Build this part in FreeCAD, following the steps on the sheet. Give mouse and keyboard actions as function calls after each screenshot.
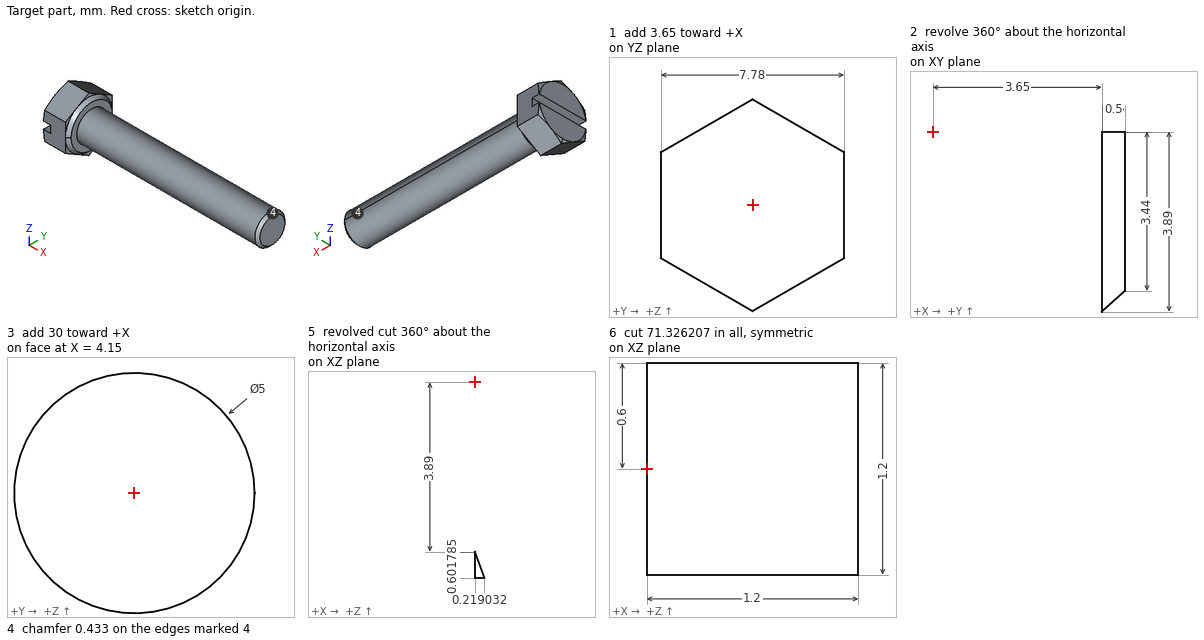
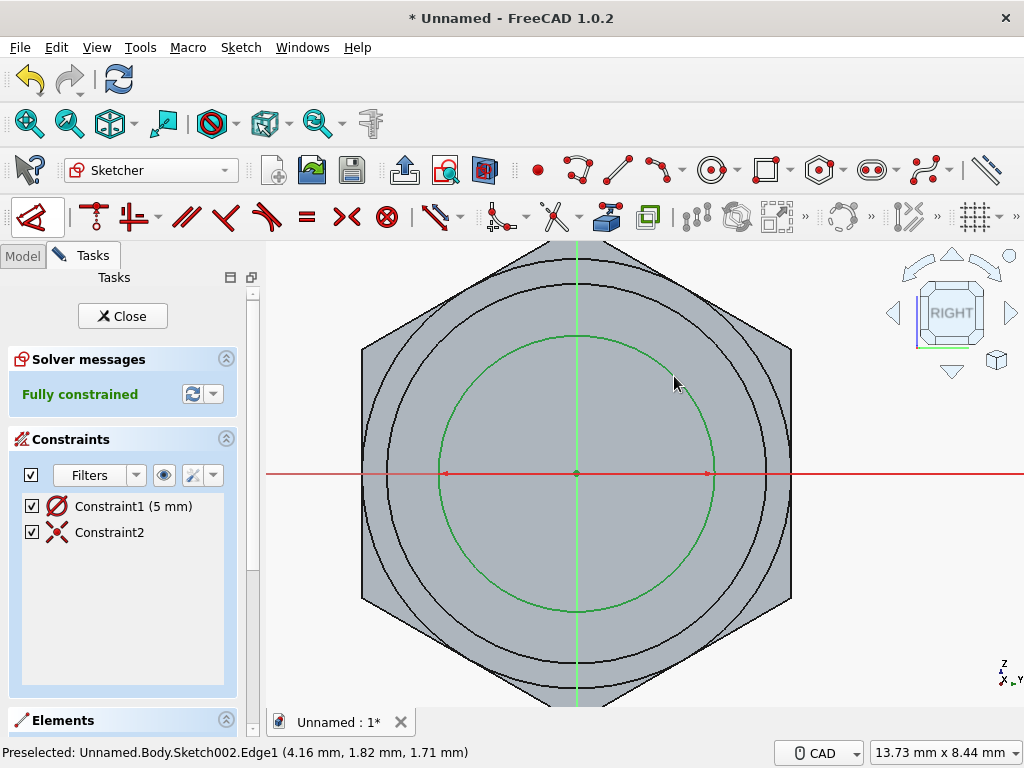
click(123, 316)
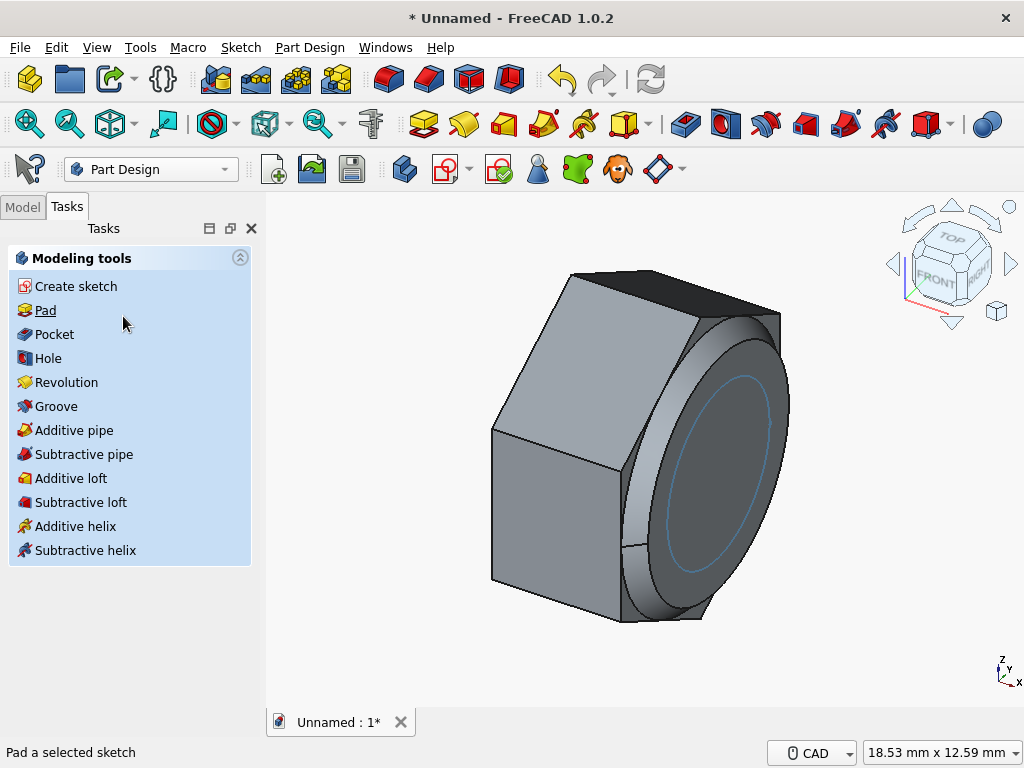
click(424, 124)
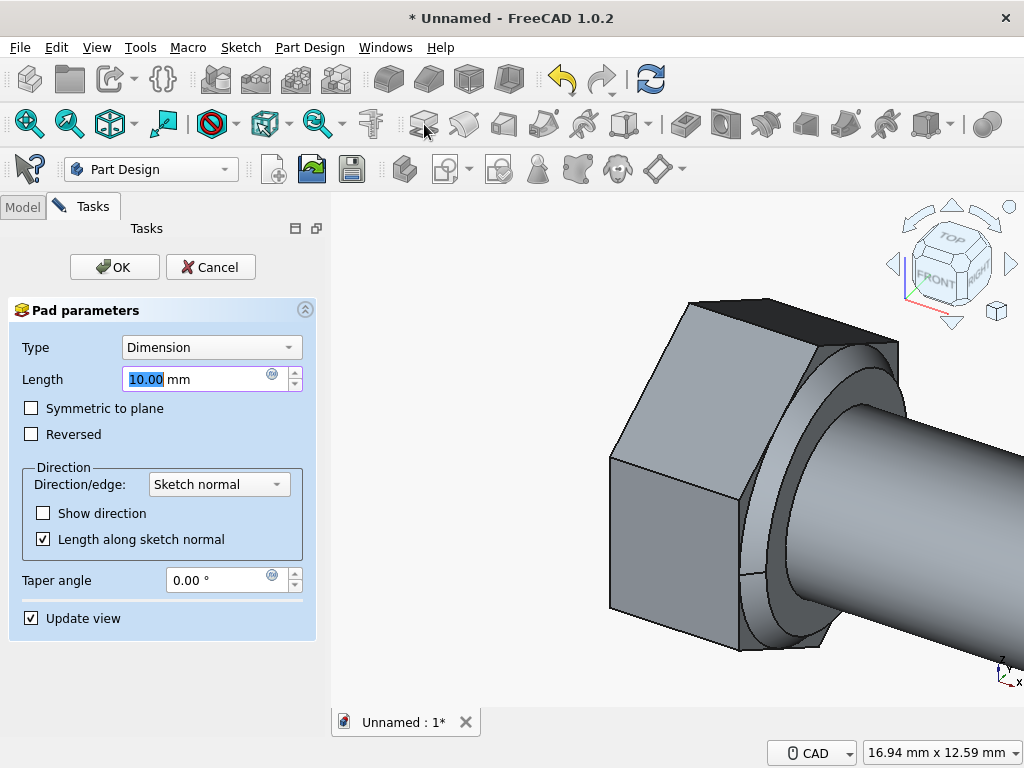
text(30)
key(Tab)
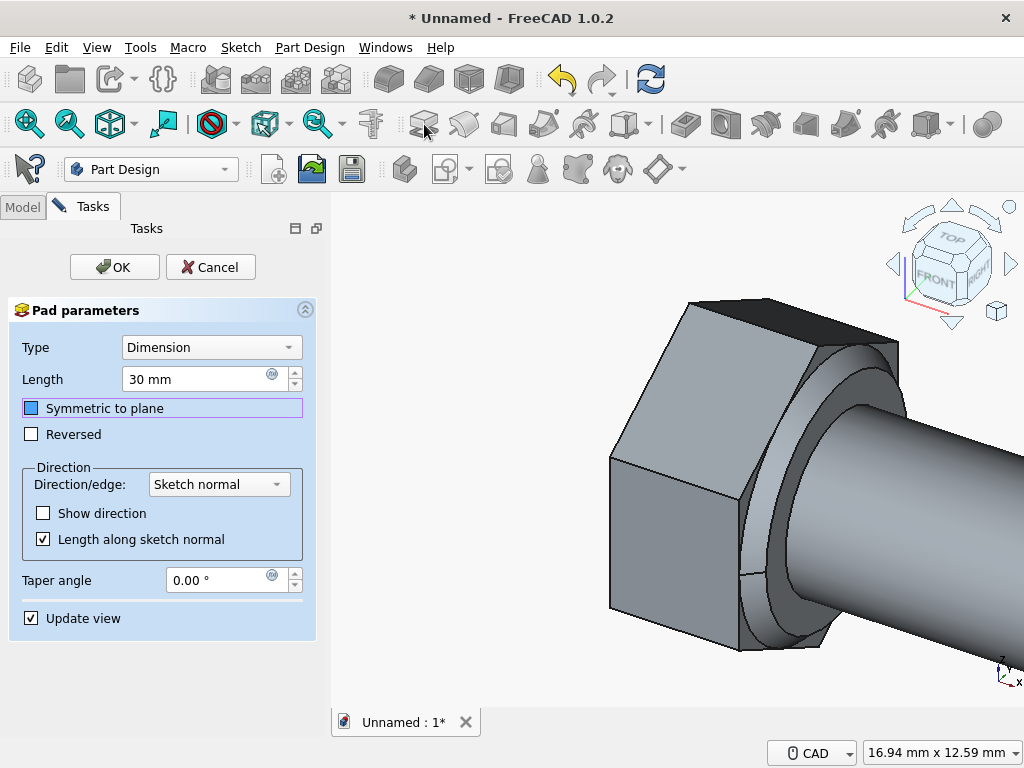
click(115, 267)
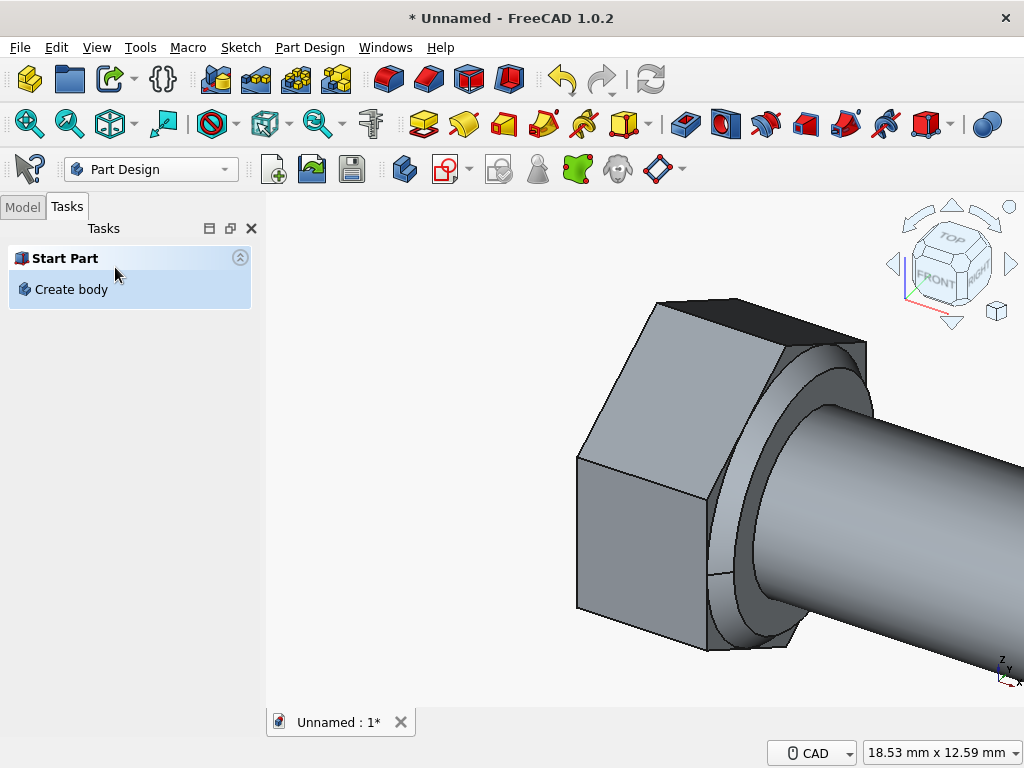
key(v)
key(f)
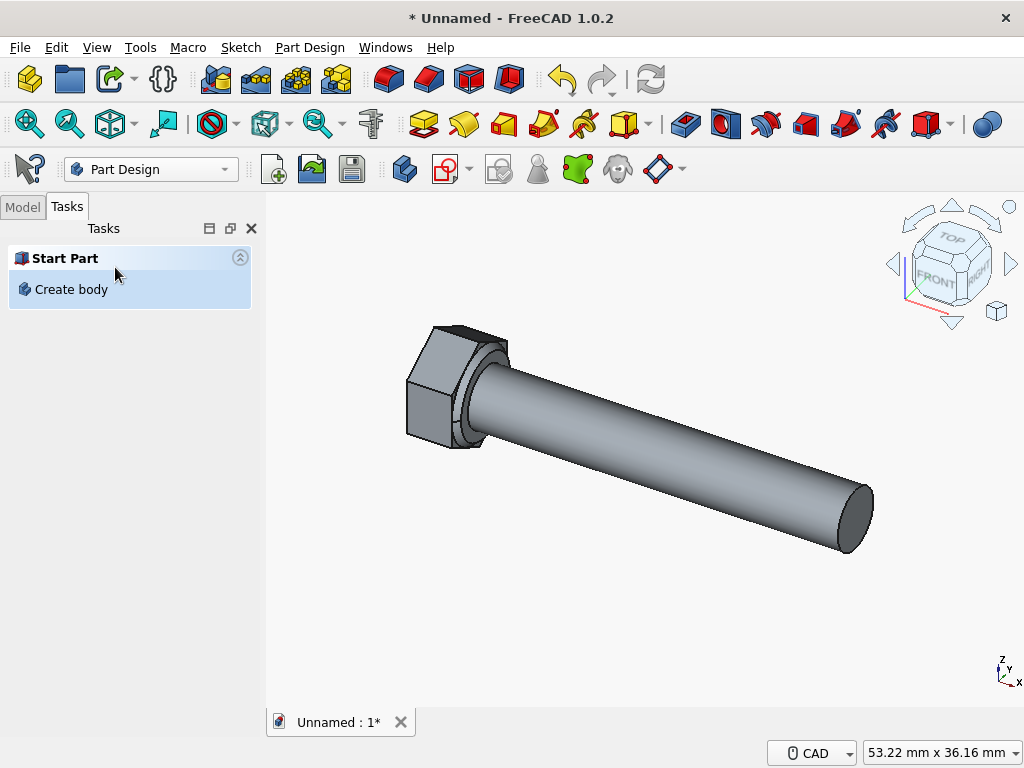
click(838, 536)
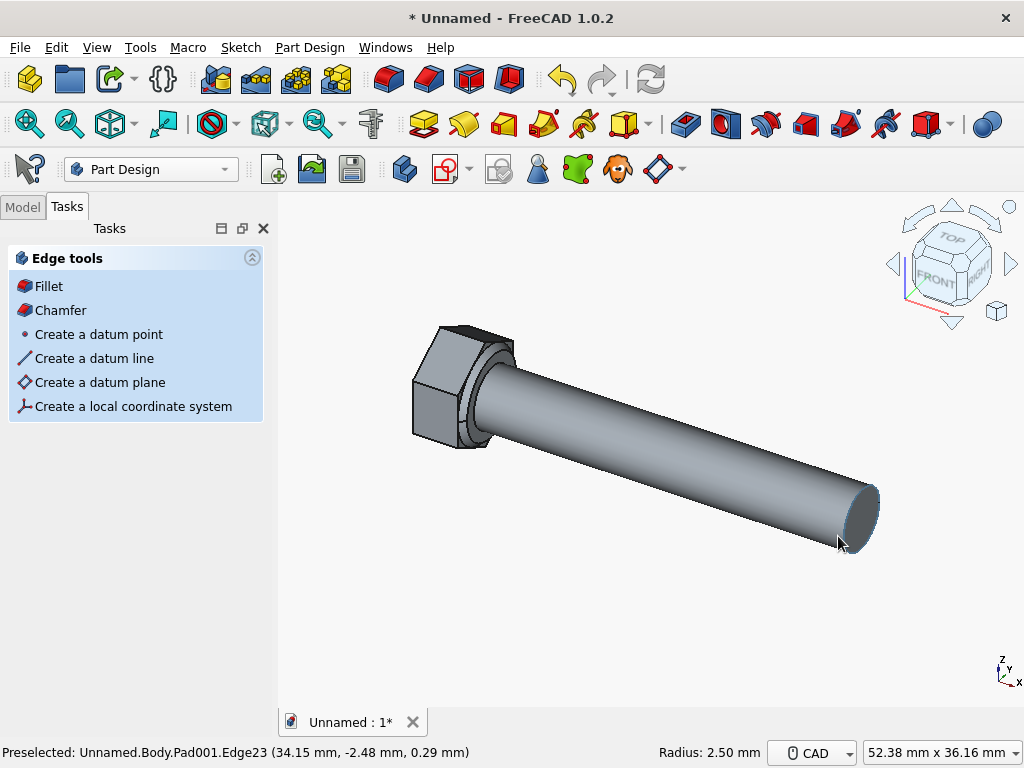
click(430, 80)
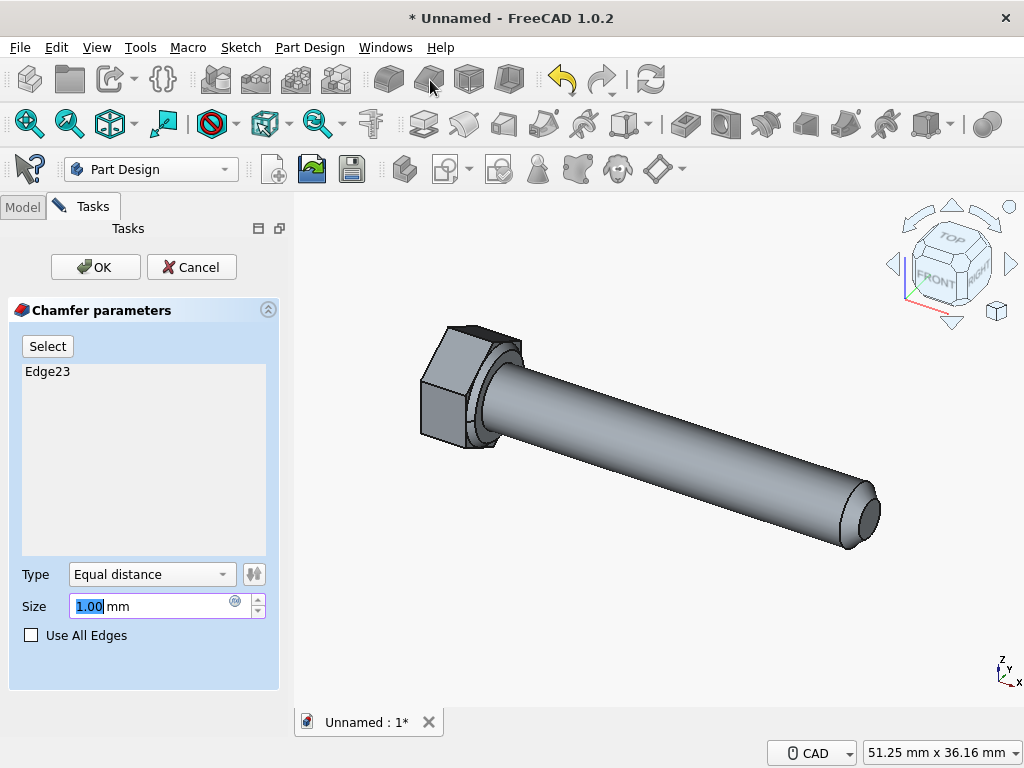
text(0.433)
key(Tab)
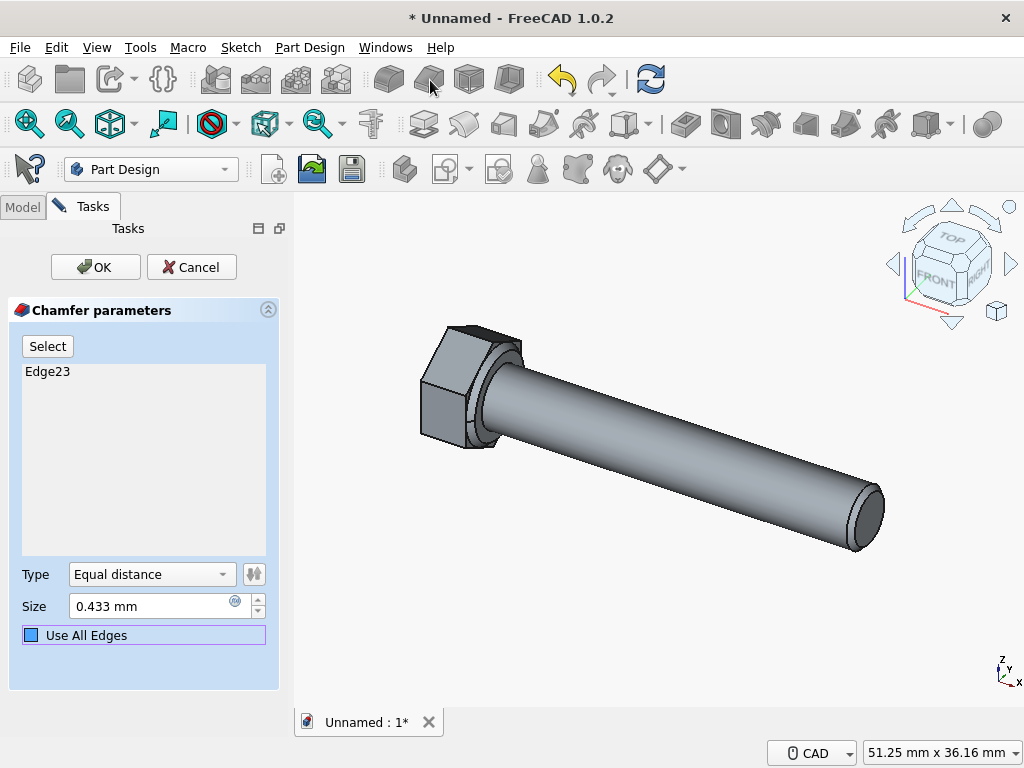
click(96, 267)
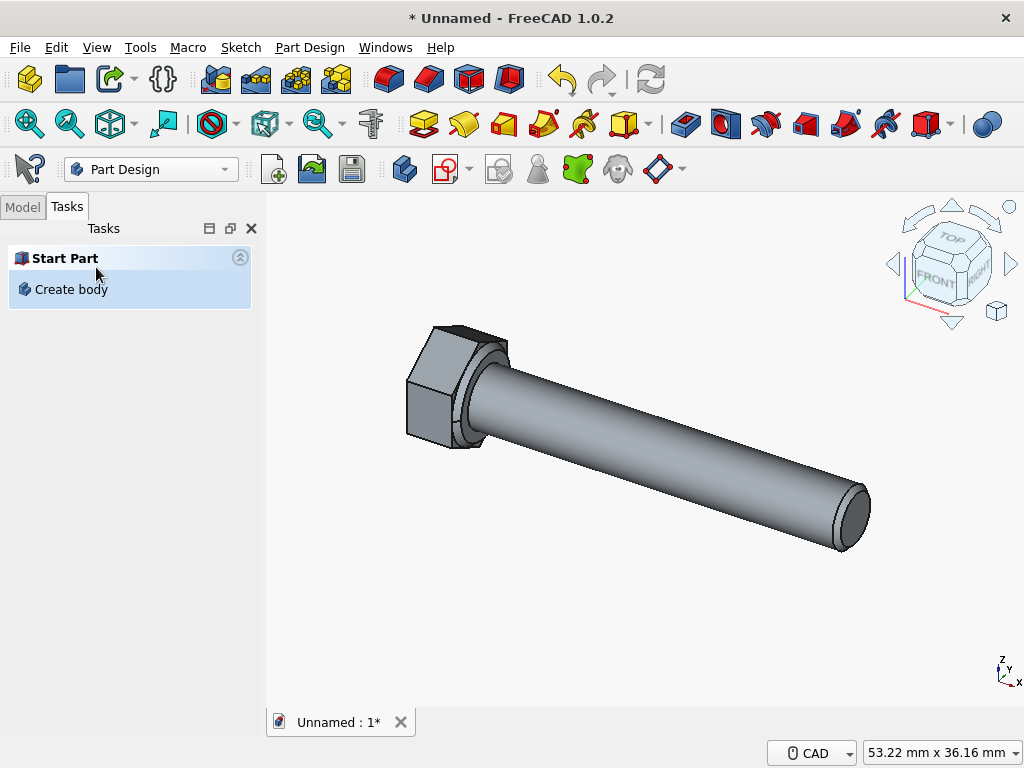
click(446, 170)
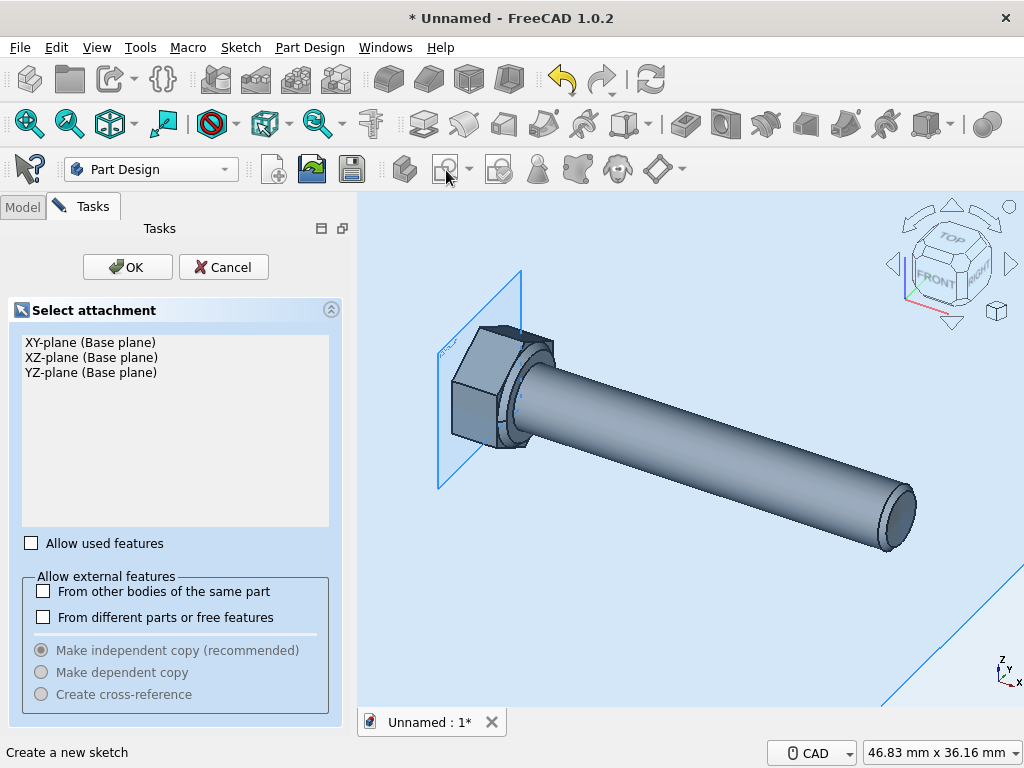
click(82, 358)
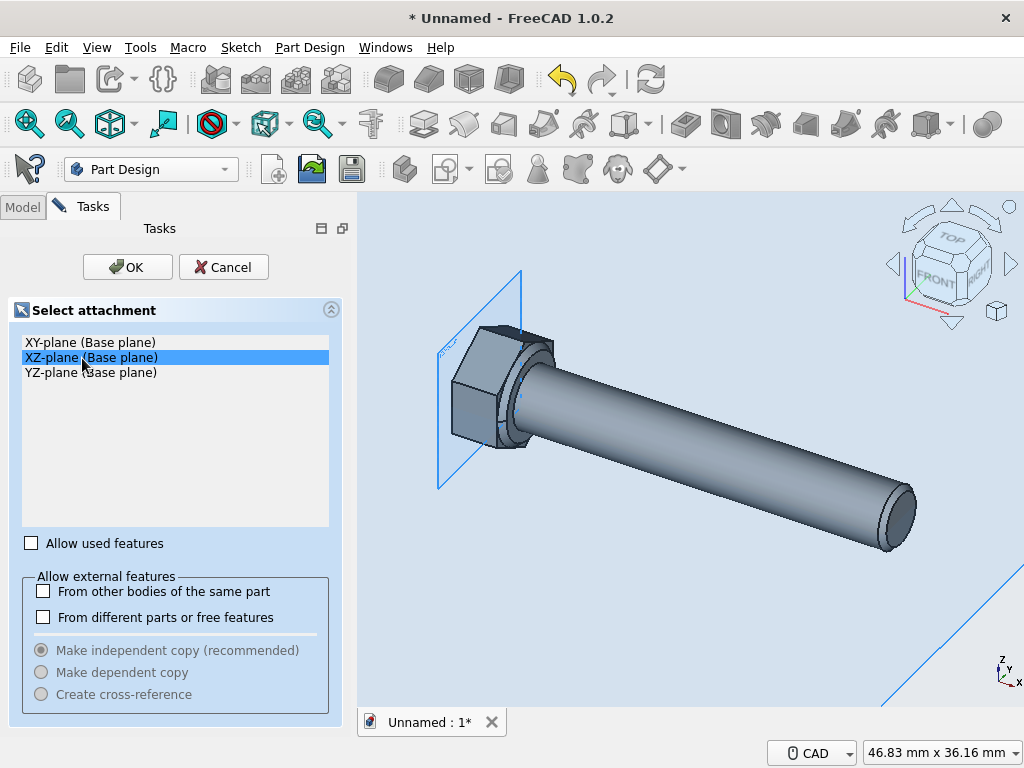
click(128, 267)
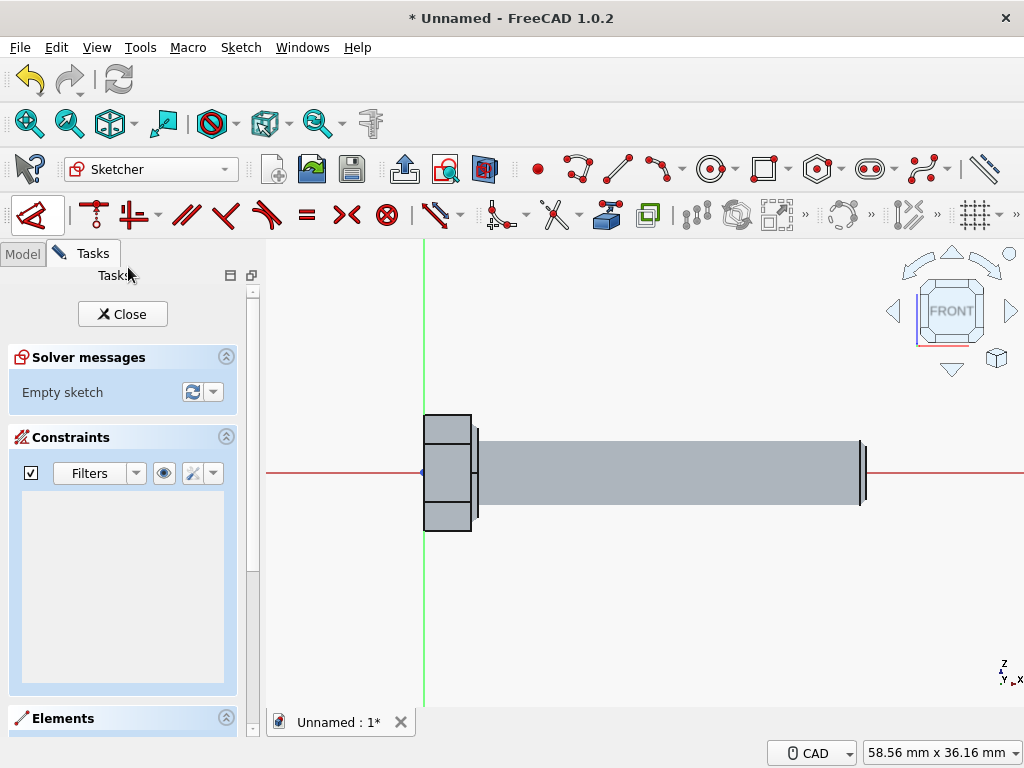
key(q)
key(s)